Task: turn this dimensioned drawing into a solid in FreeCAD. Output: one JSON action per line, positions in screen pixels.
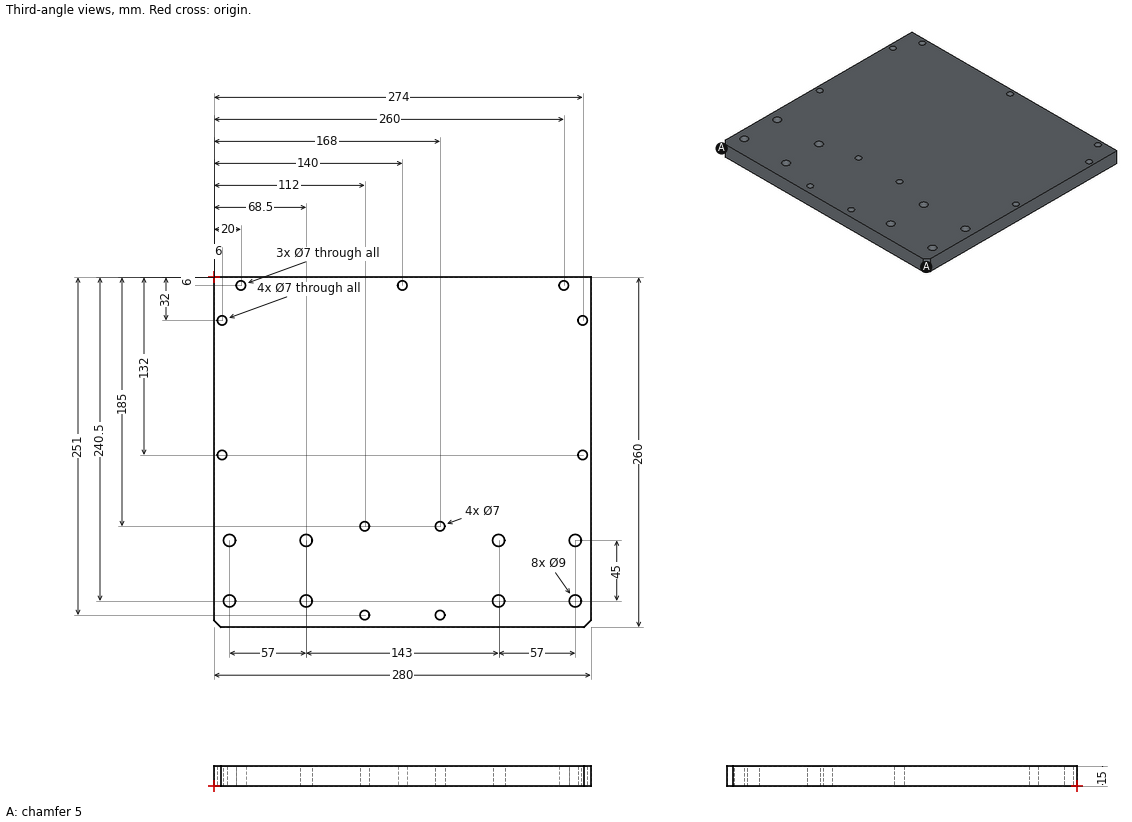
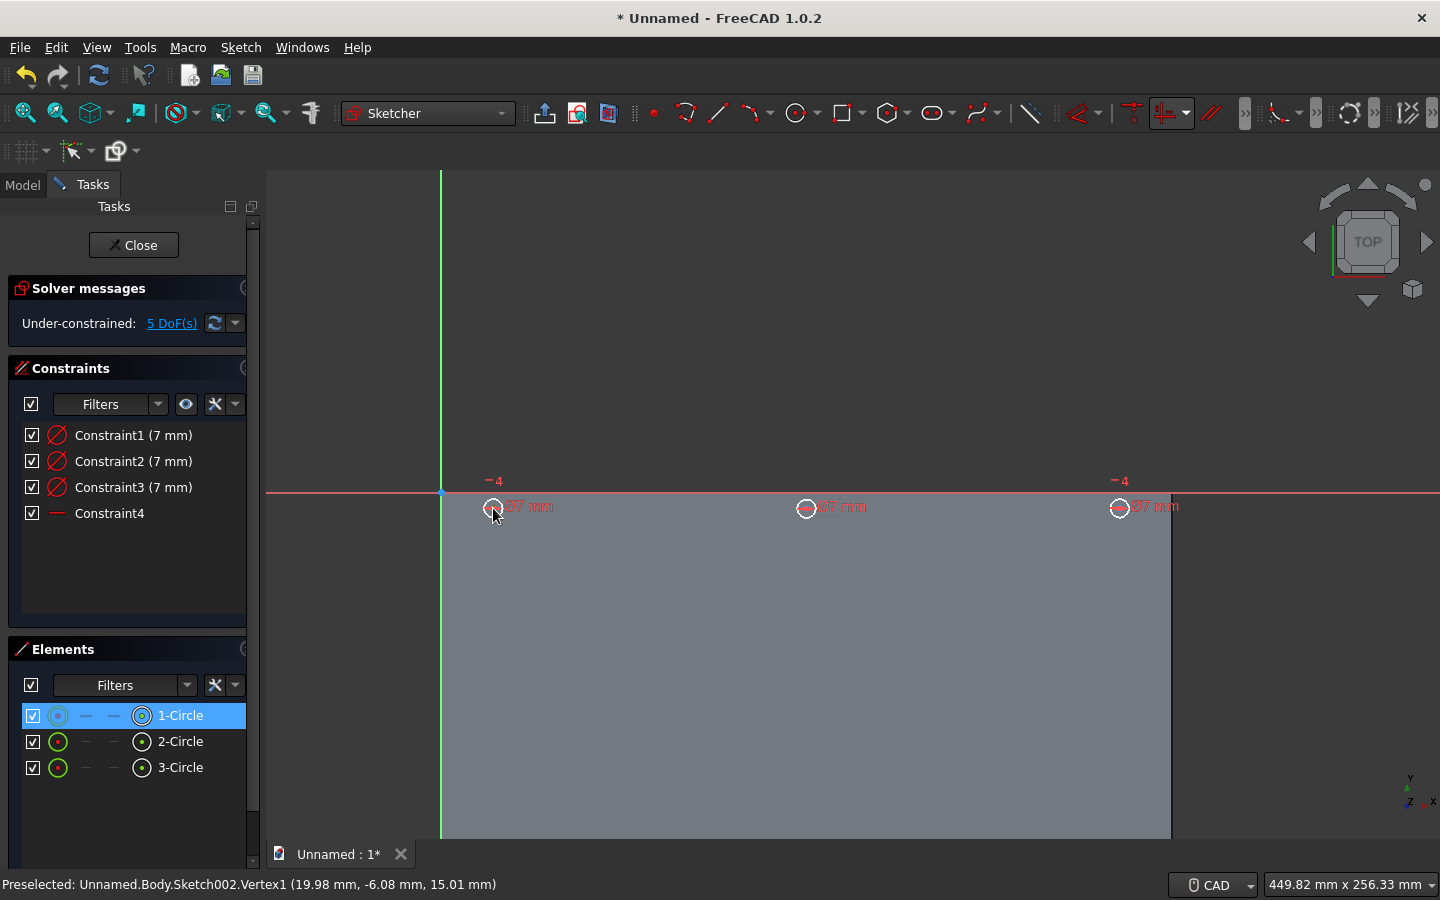
{"action": "left_click", "coordinate": [807, 509]}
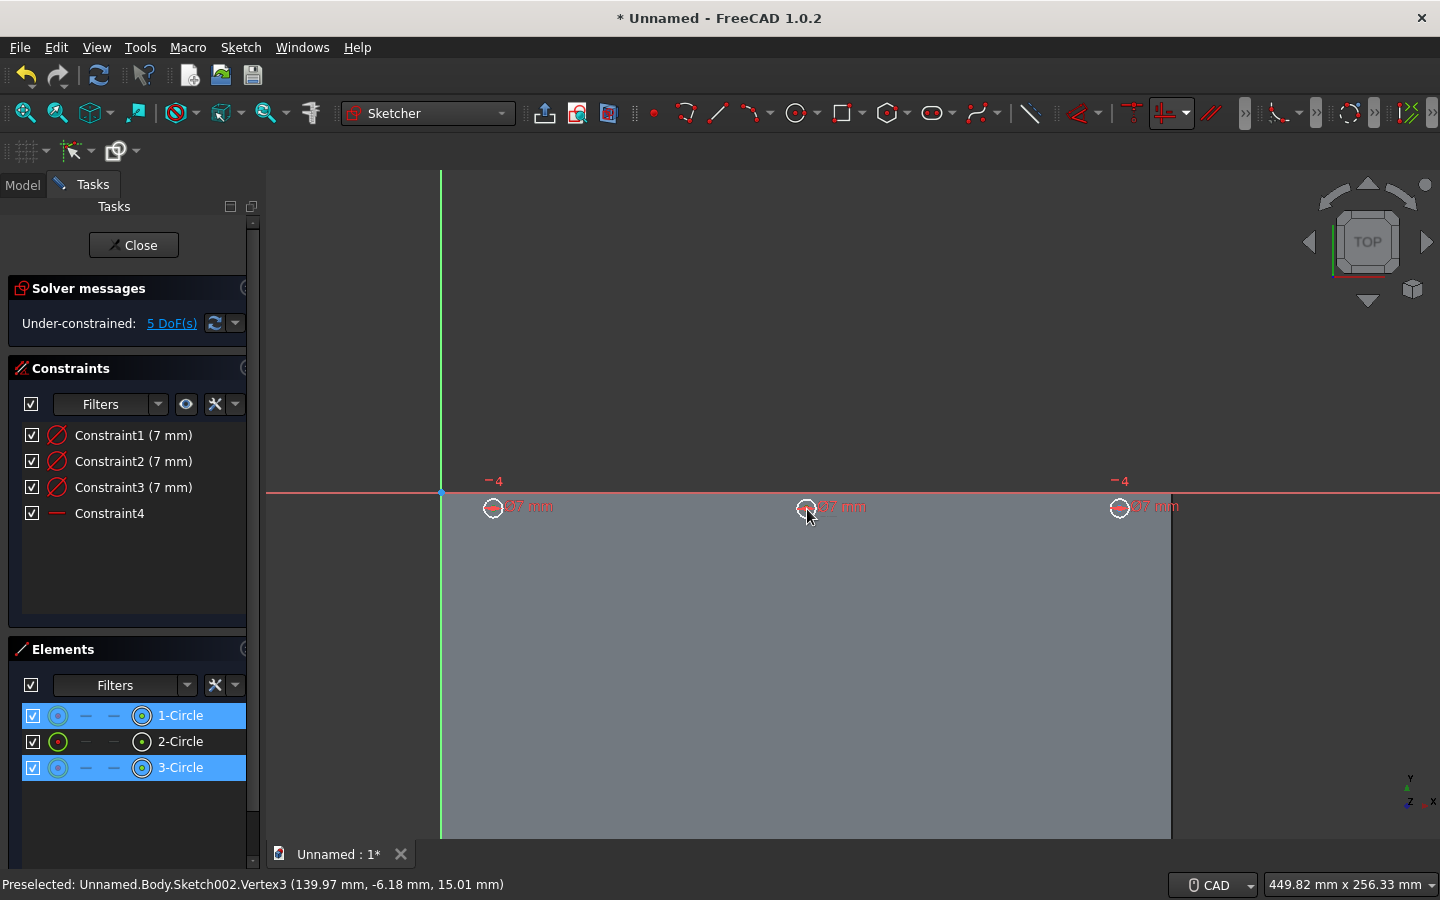
{"action": "left_click", "coordinate": [1188, 114]}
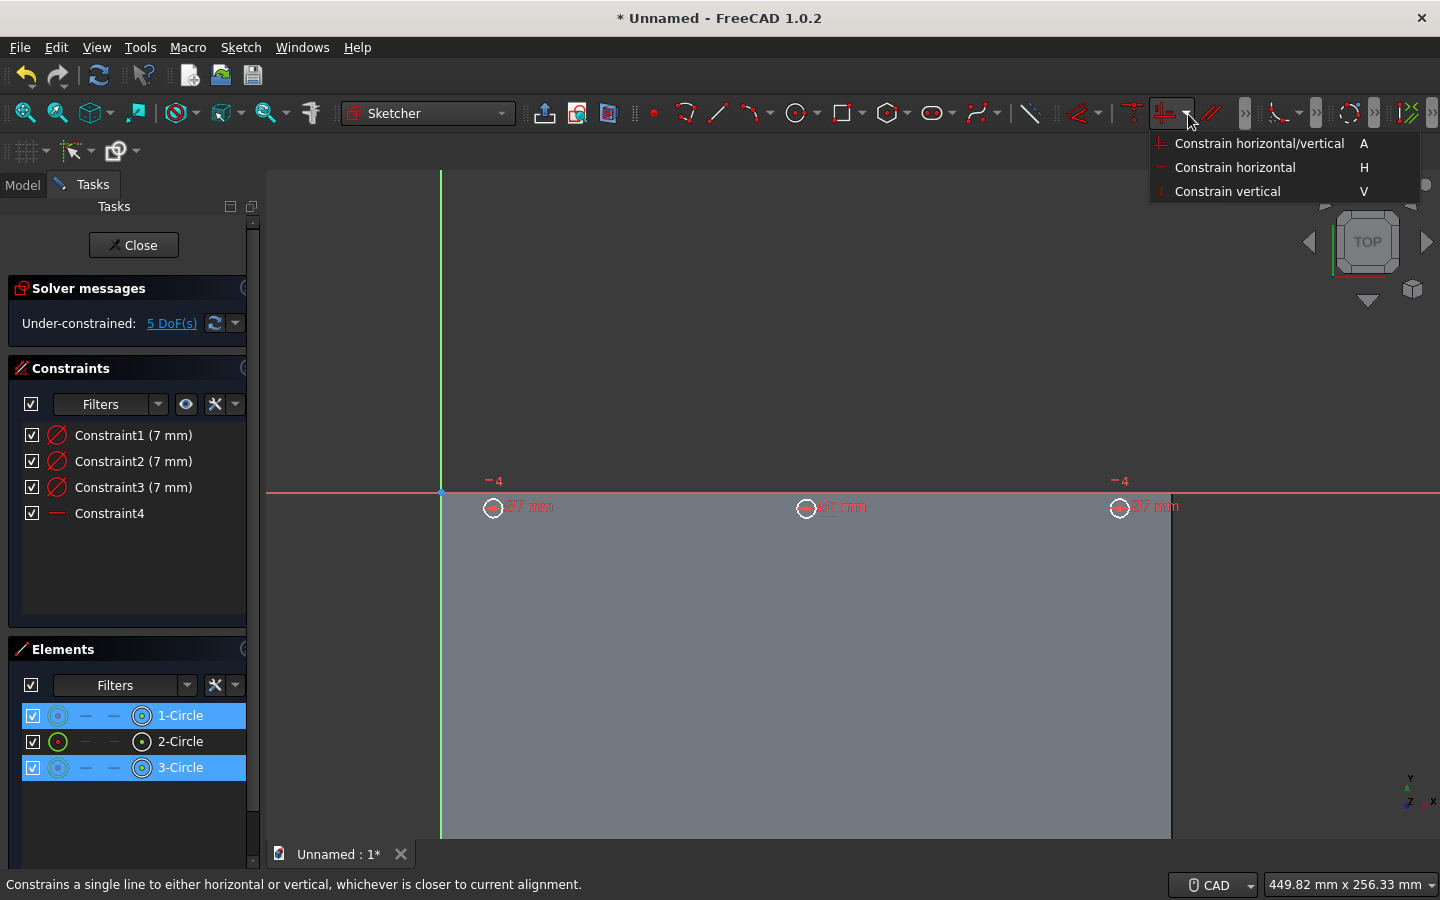
{"action": "left_click", "coordinate": [1285, 167]}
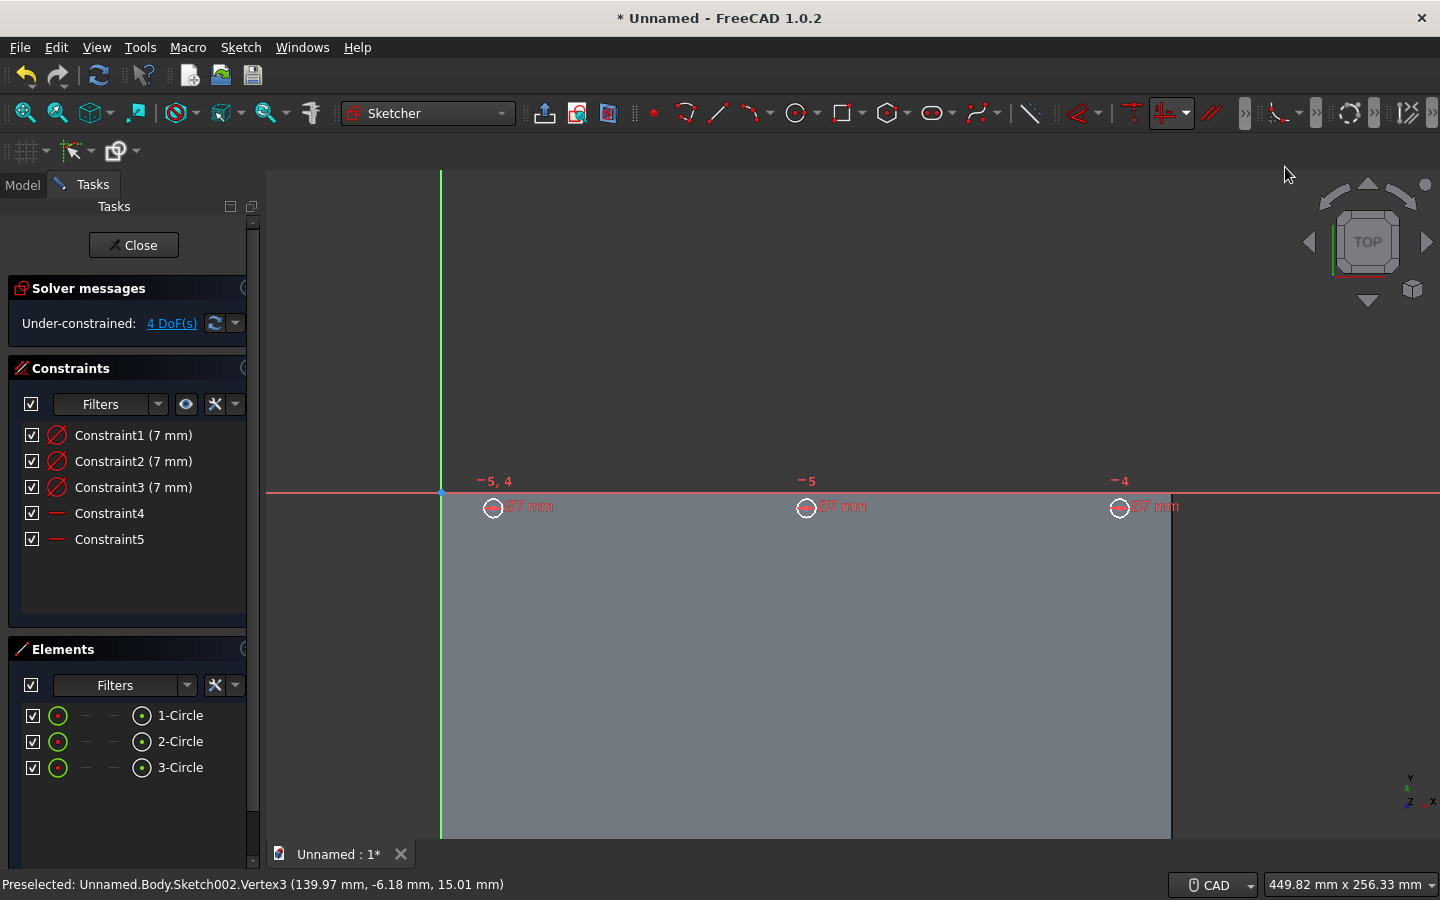
{"action": "left_click", "coordinate": [1078, 114]}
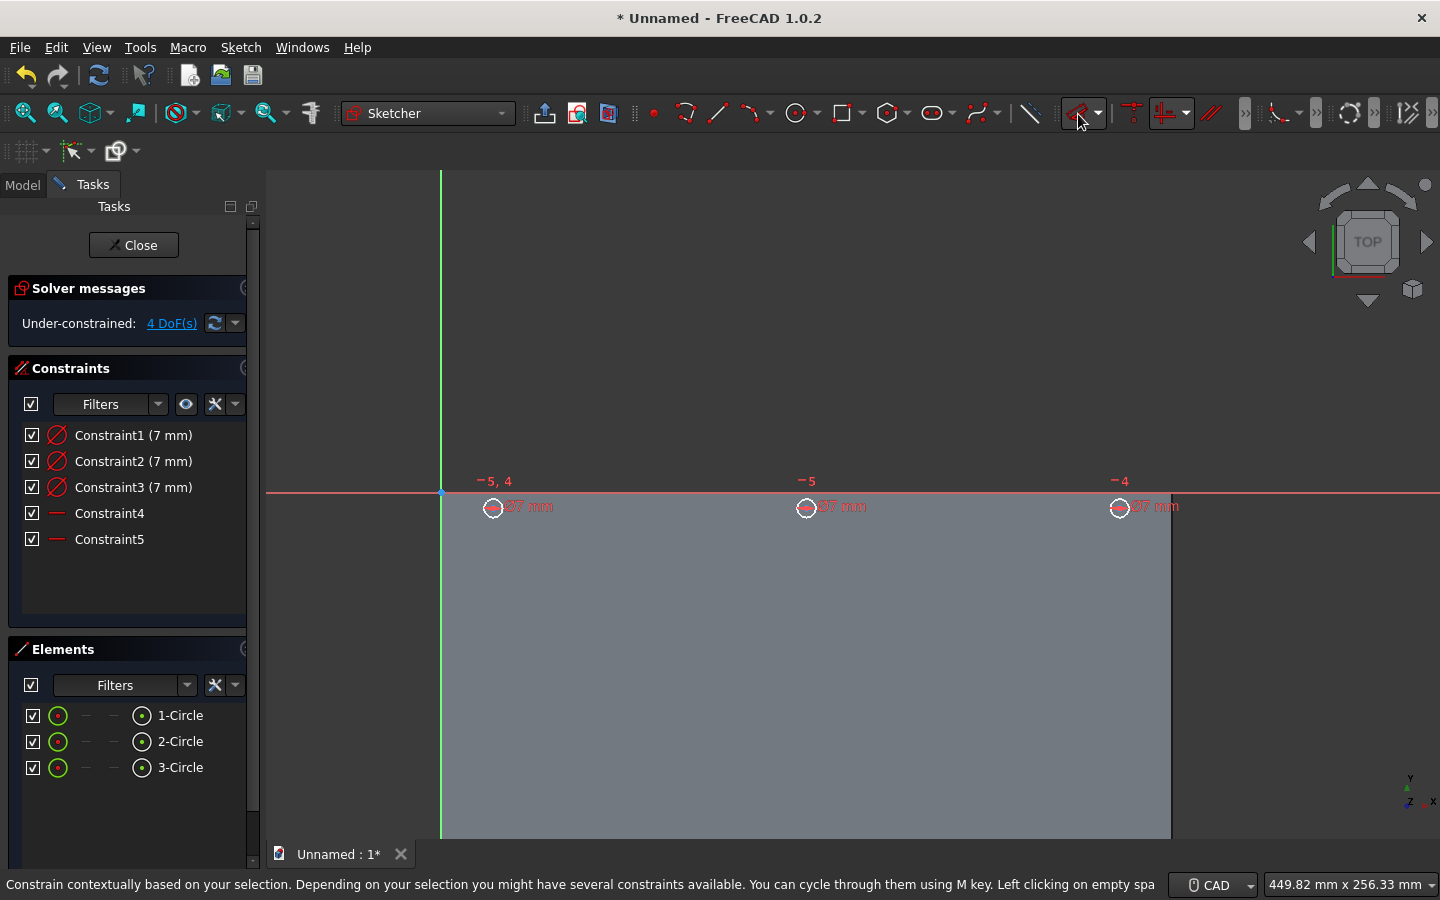
{"action": "scroll", "coordinate": [493, 508], "scroll_direction": "up", "scroll_amount": 5}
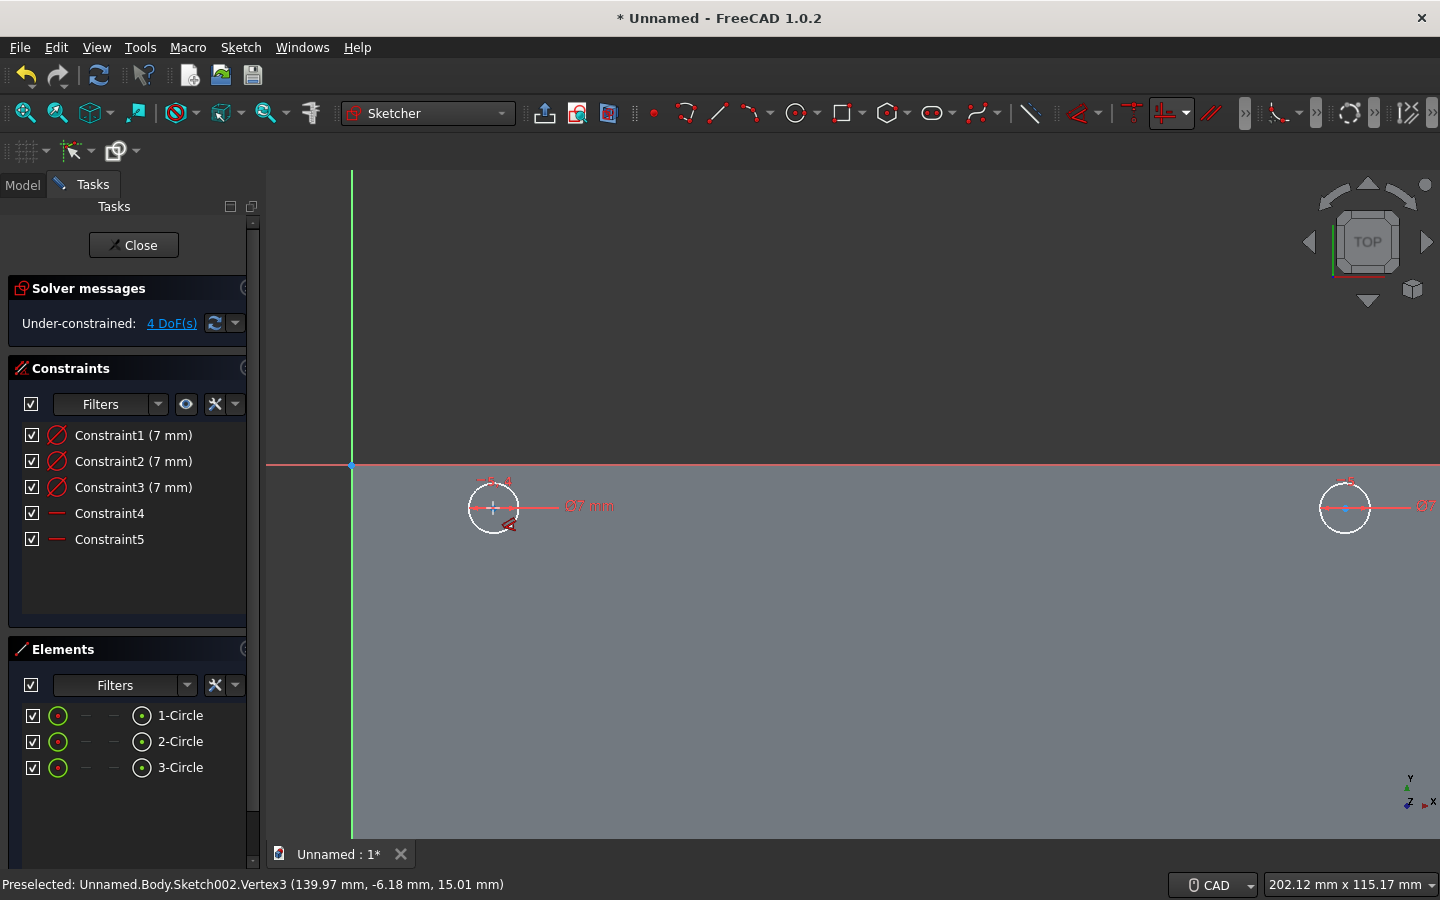
{"action": "left_click", "coordinate": [494, 508]}
{"action": "left_click", "coordinate": [318, 487]}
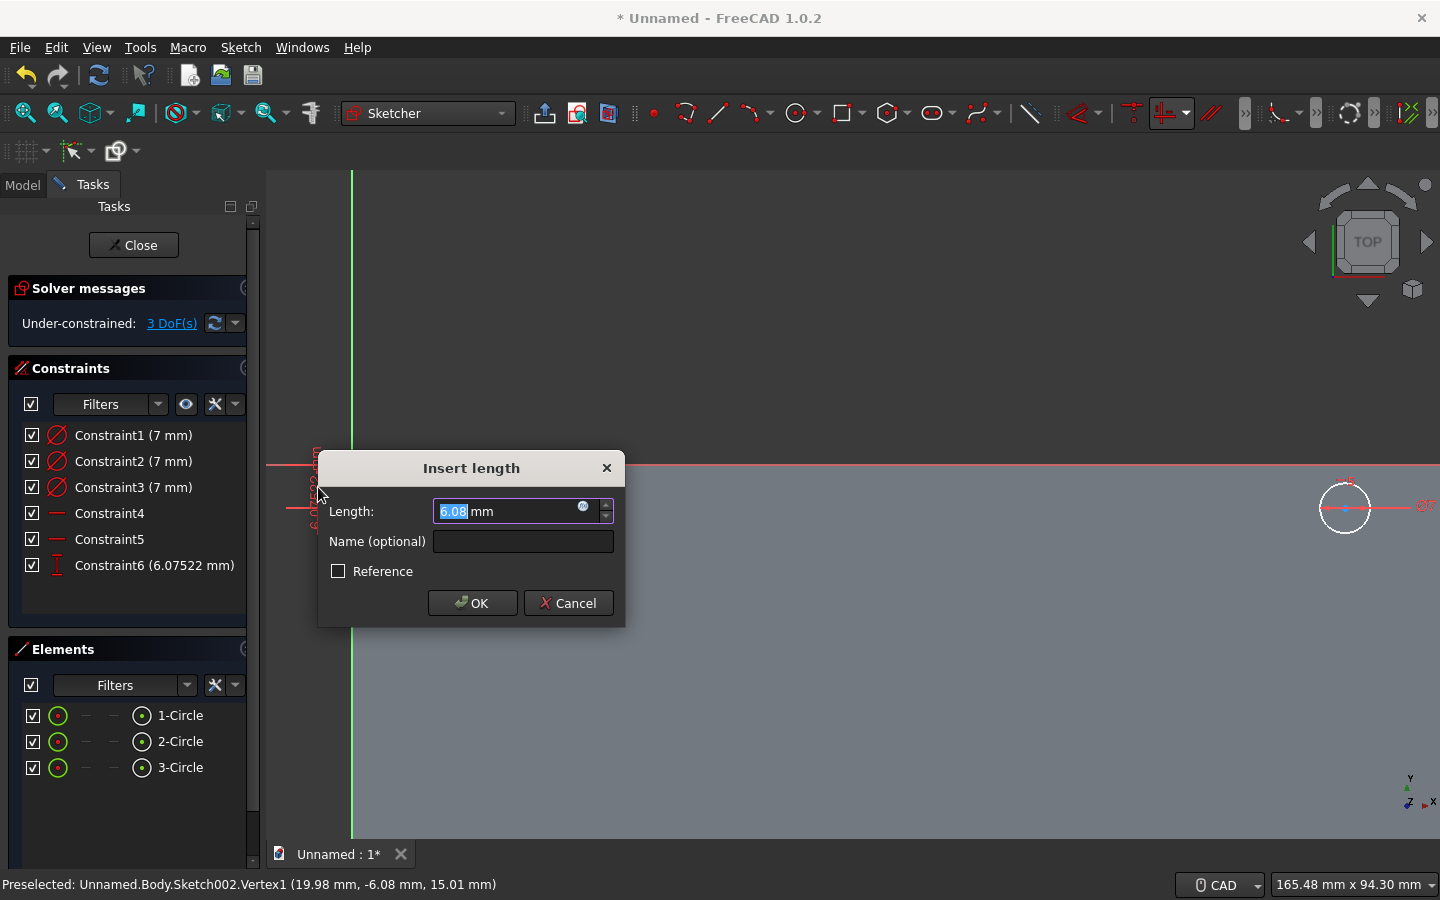
{"action": "type", "text": "6"}
{"action": "key", "text": "Return"}